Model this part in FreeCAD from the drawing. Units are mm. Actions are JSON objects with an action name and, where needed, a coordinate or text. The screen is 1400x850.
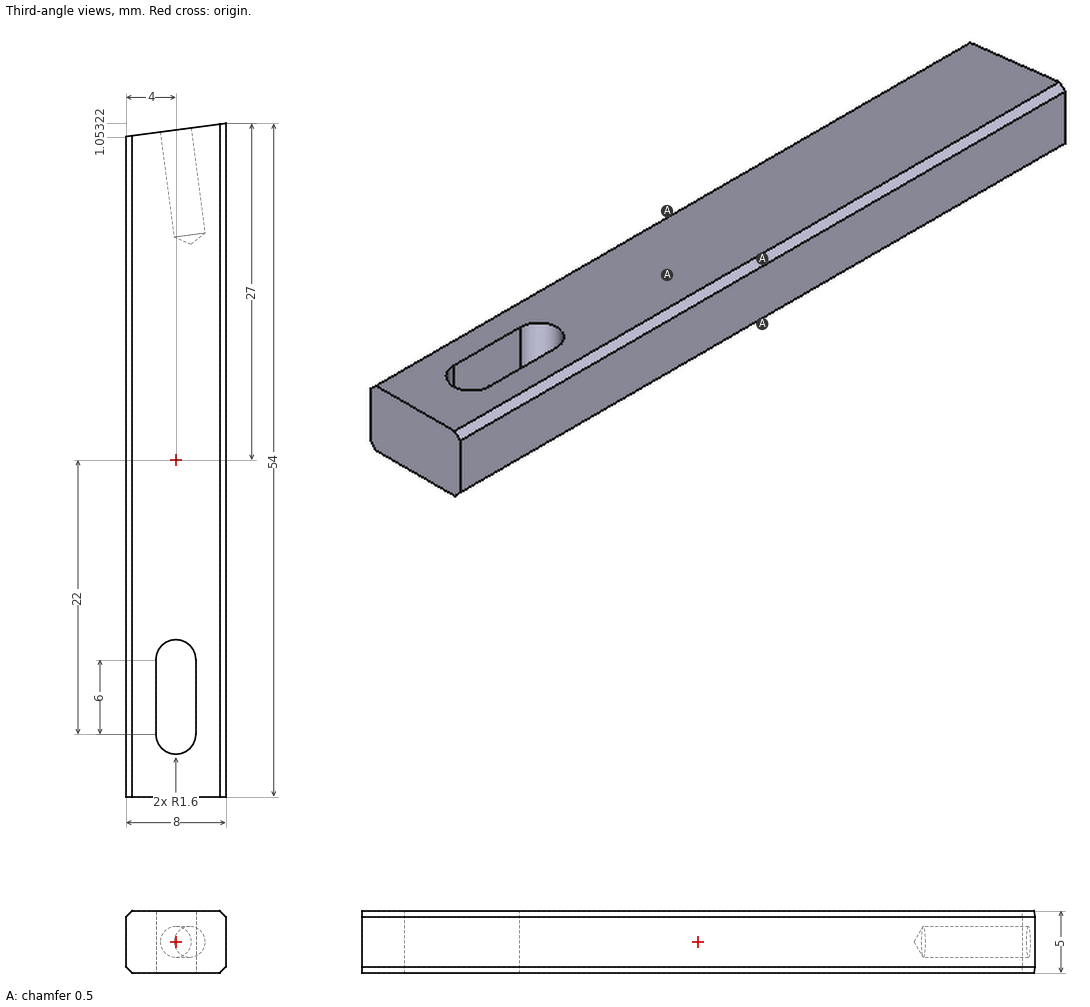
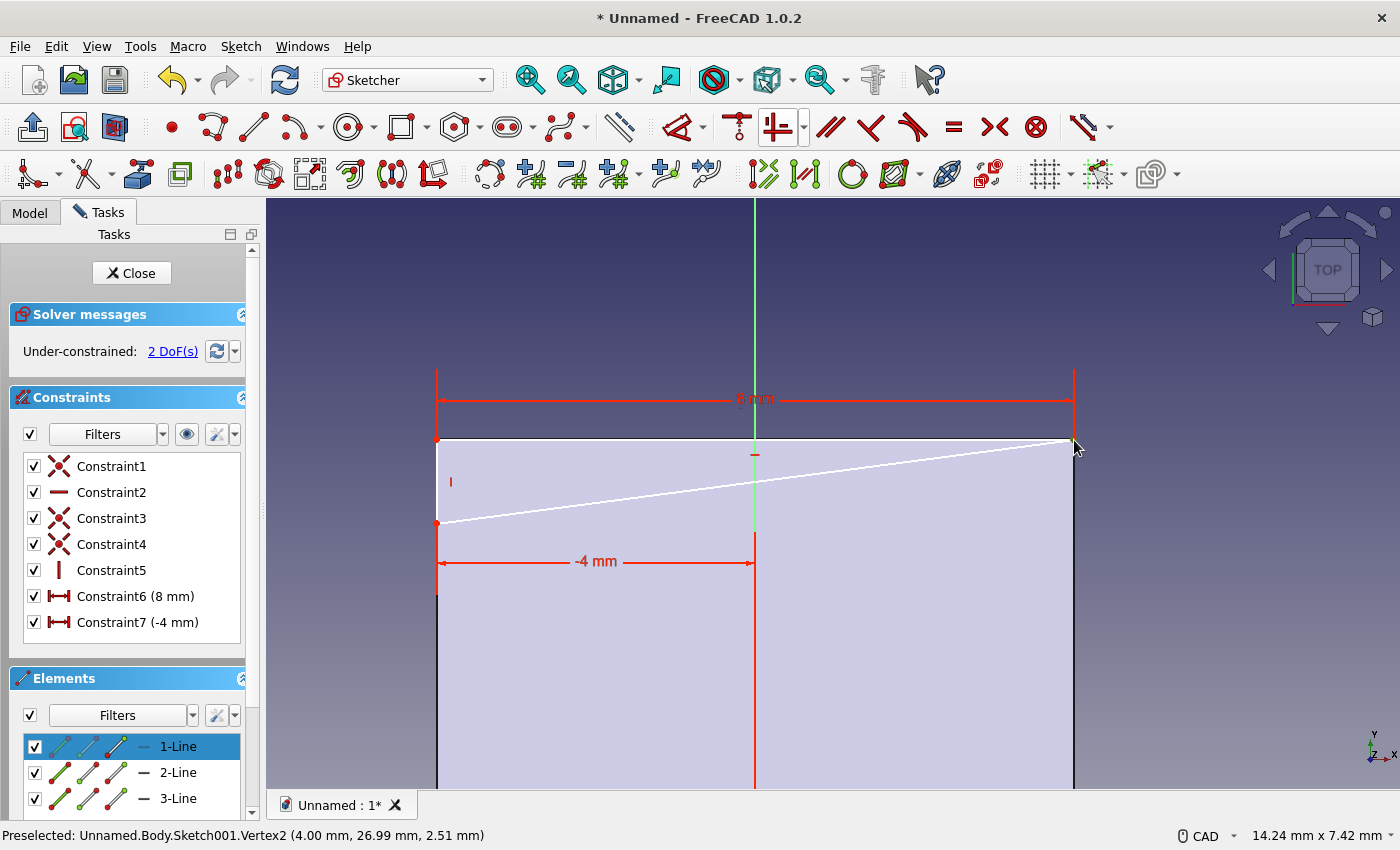
{"action": "key", "text": "i"}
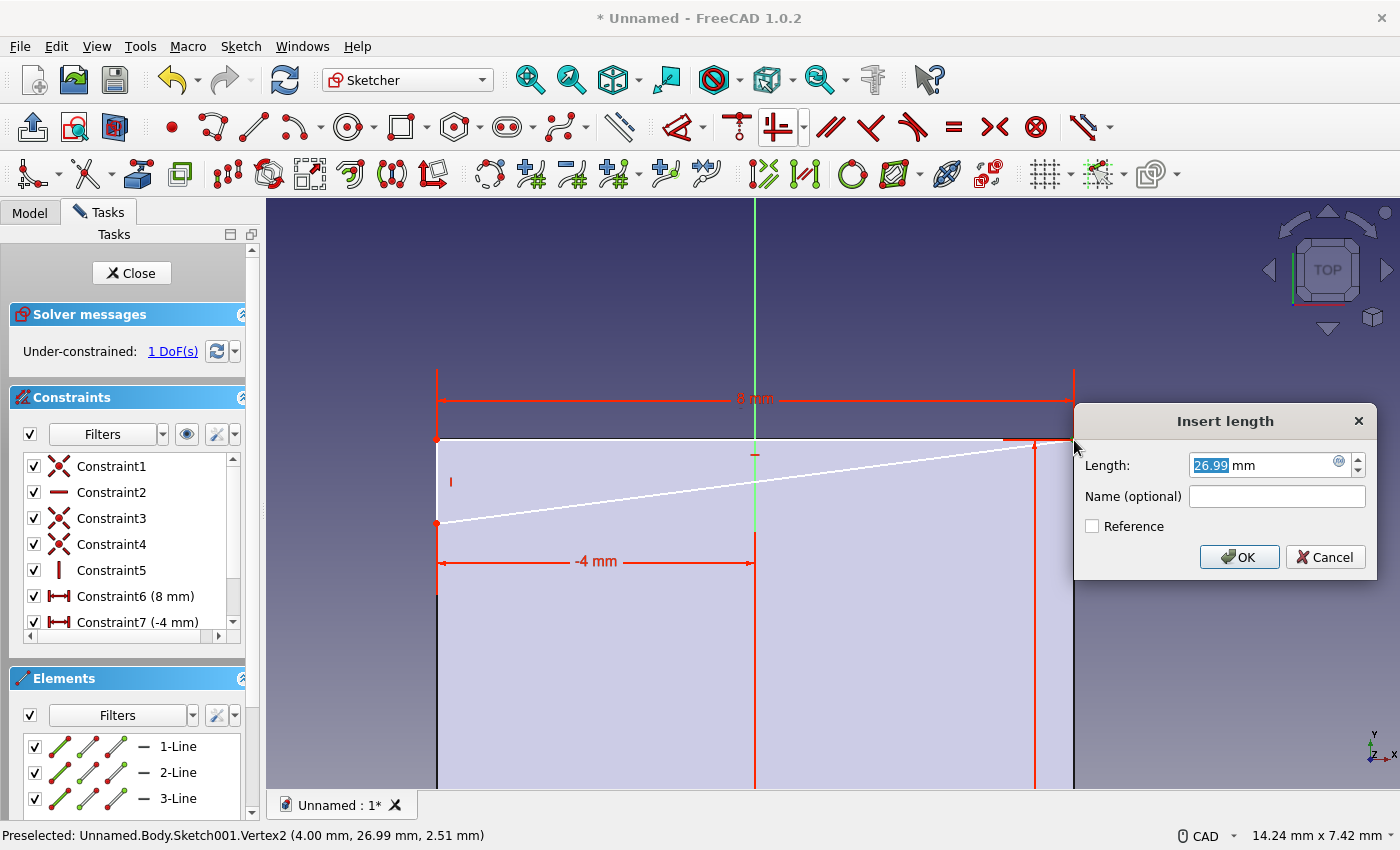
{"action": "type", "text": "27"}
{"action": "key", "text": "Return"}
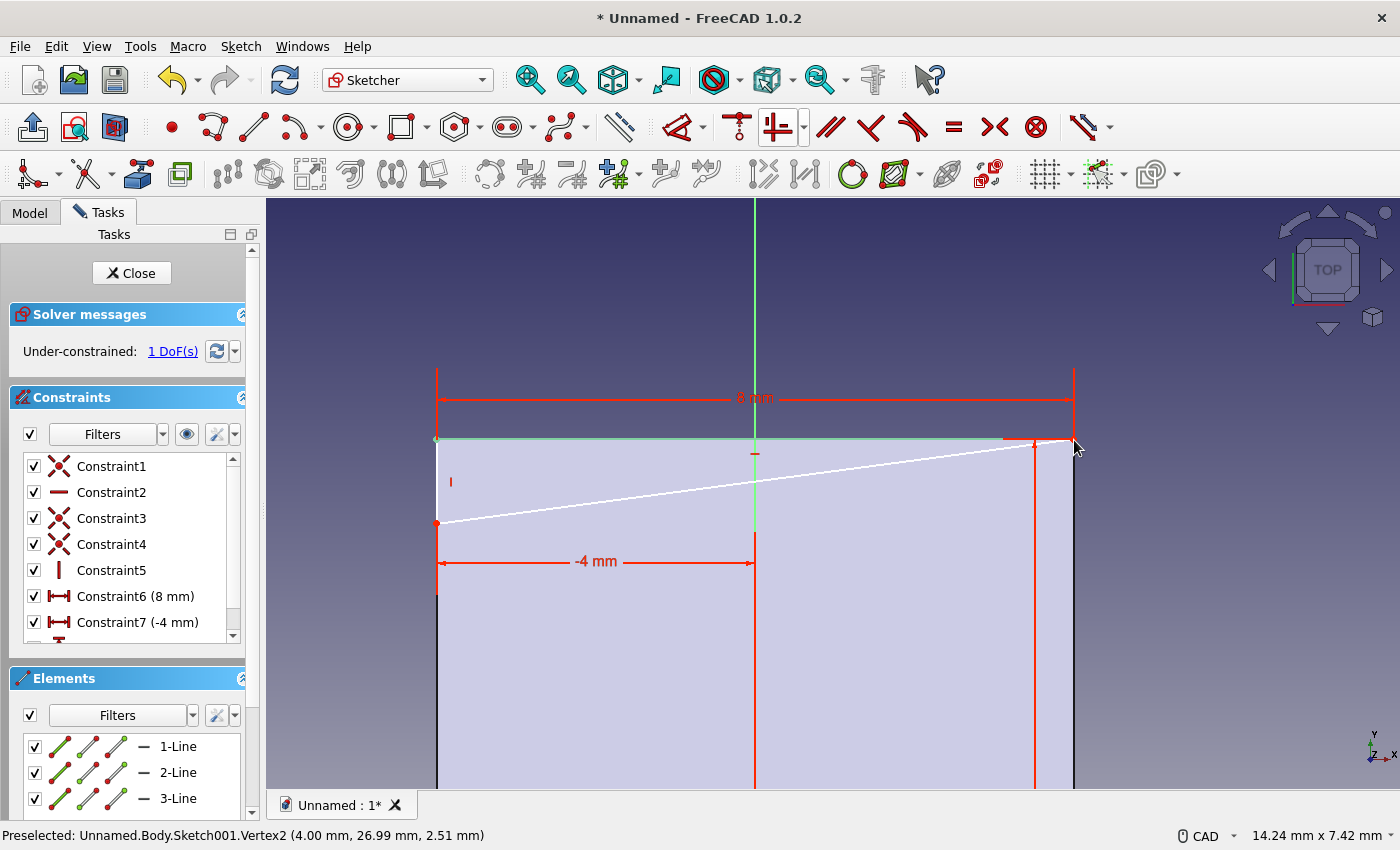
{"action": "left_click", "coordinate": [437, 465]}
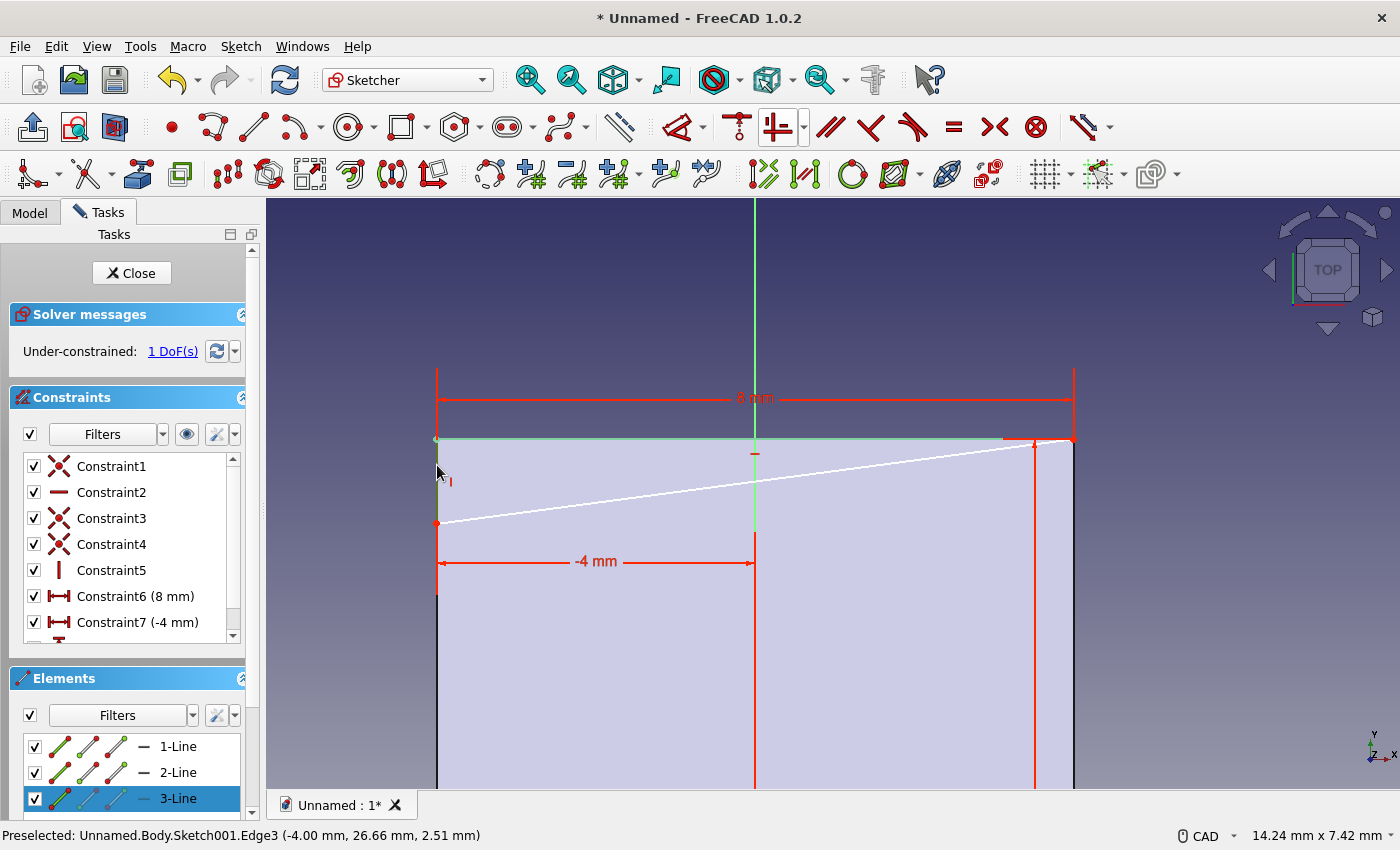
{"action": "key", "text": "i"}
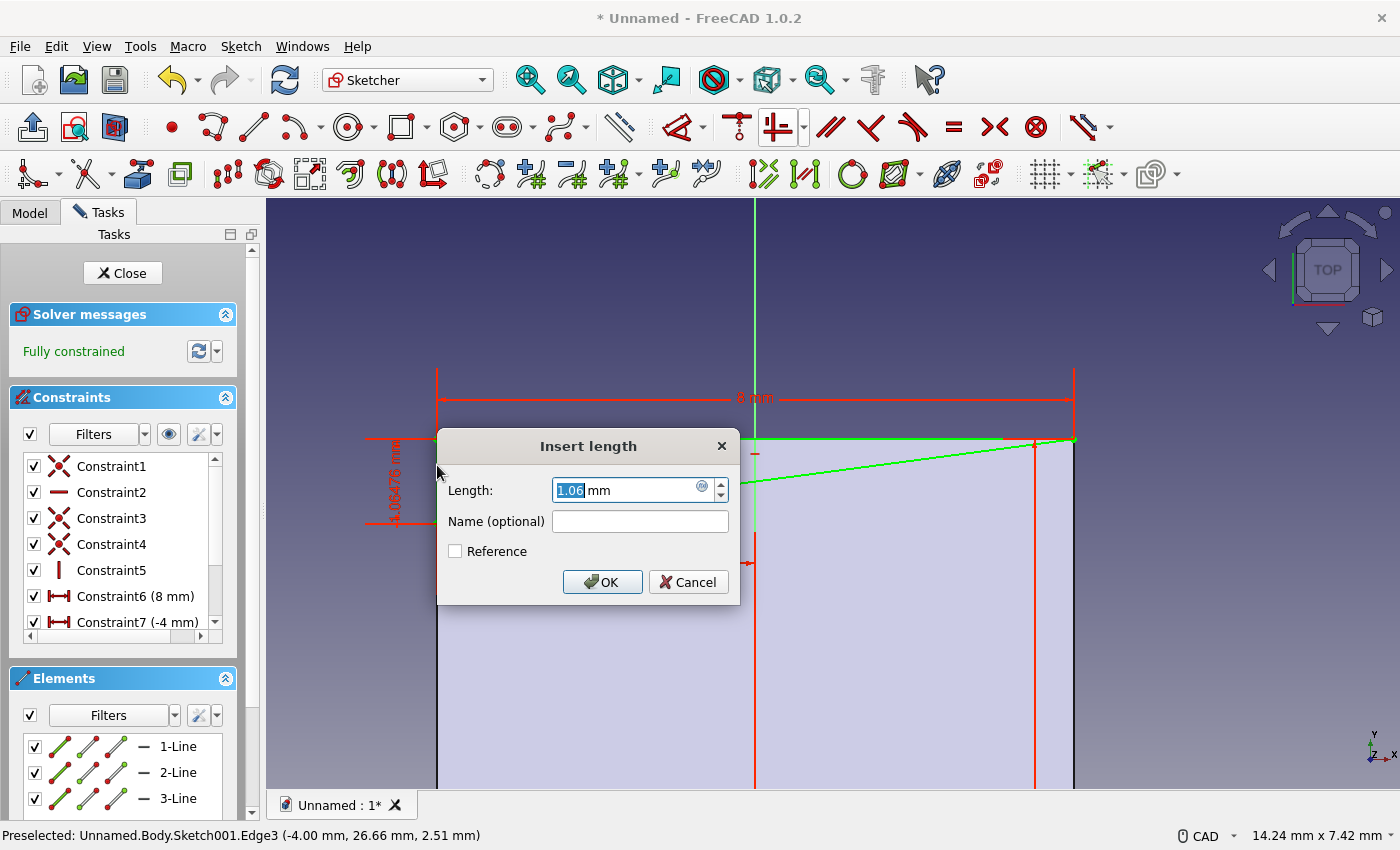
{"action": "type", "text": "1.05322"}
{"action": "key", "text": "Return"}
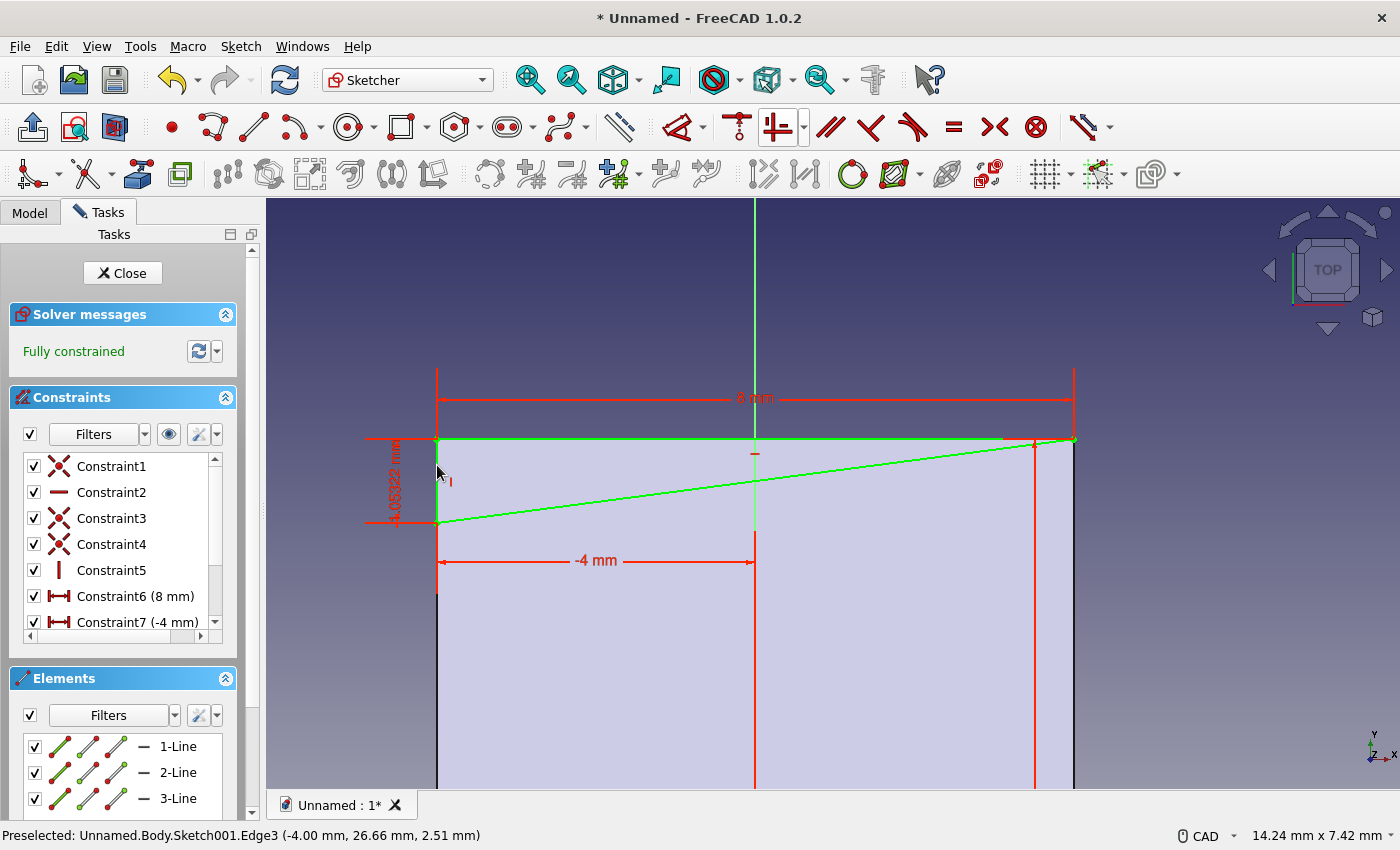
{"action": "left_click", "coordinate": [123, 273]}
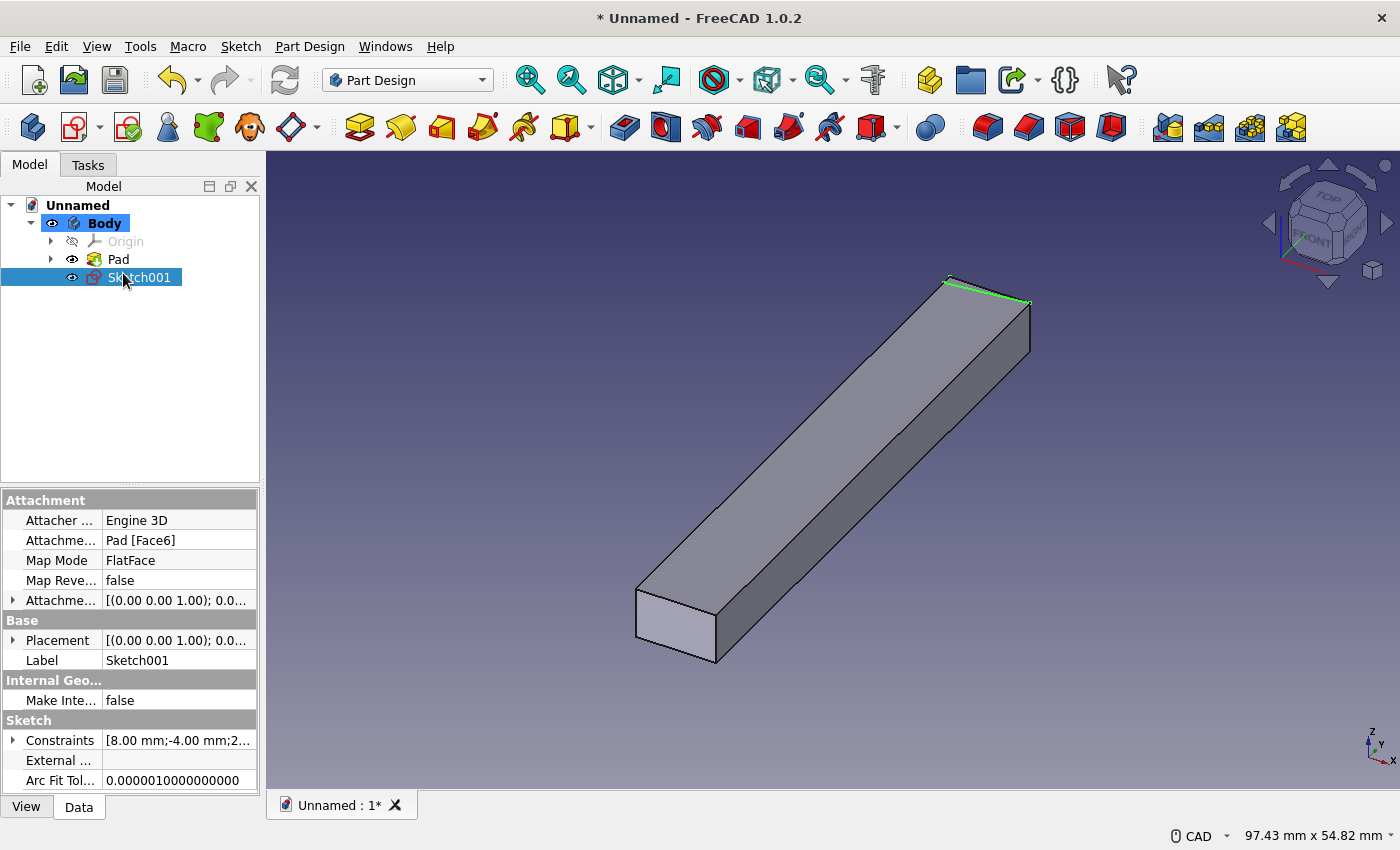
{"action": "left_click", "coordinate": [625, 128]}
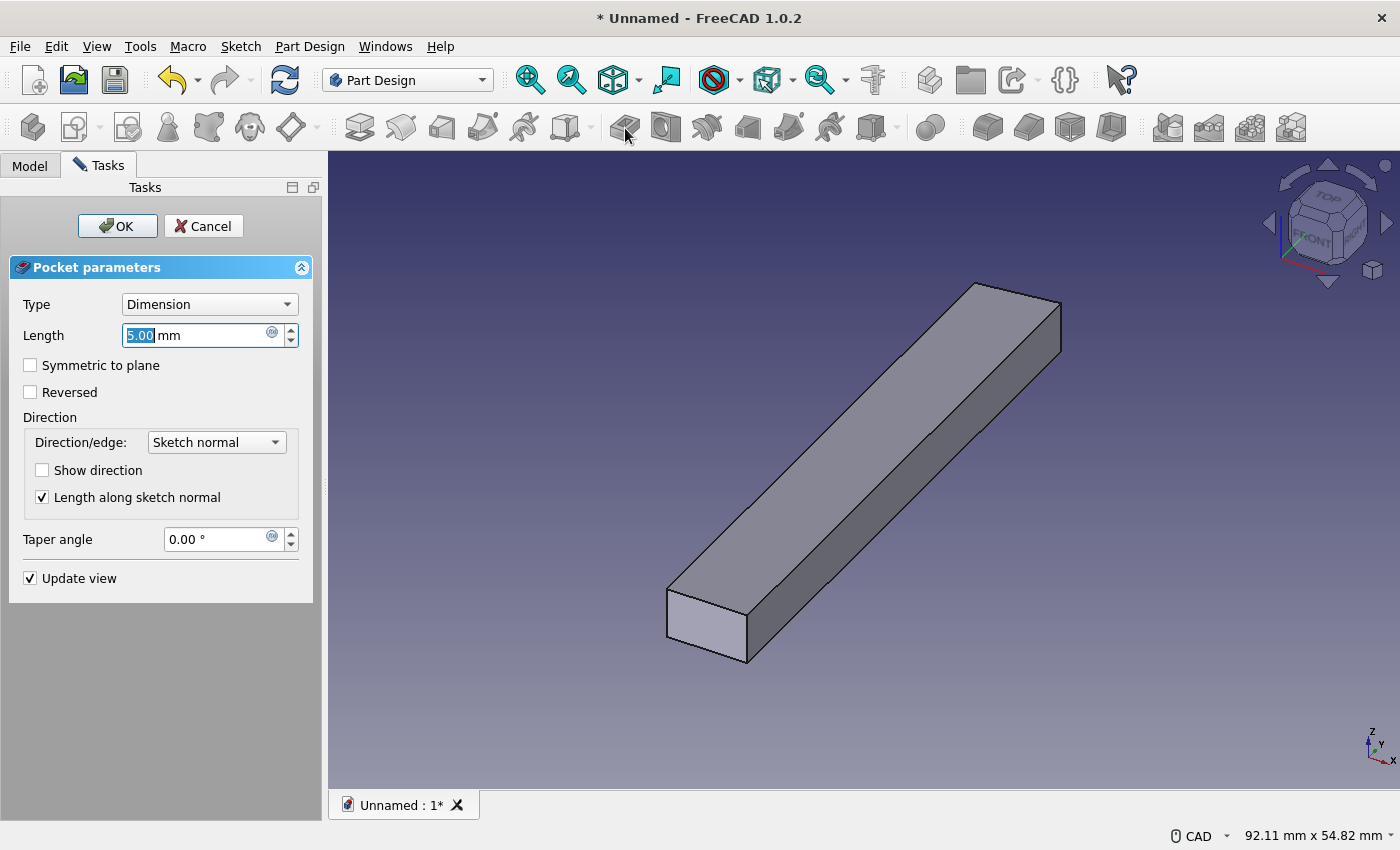
{"action": "left_click", "coordinate": [210, 304]}